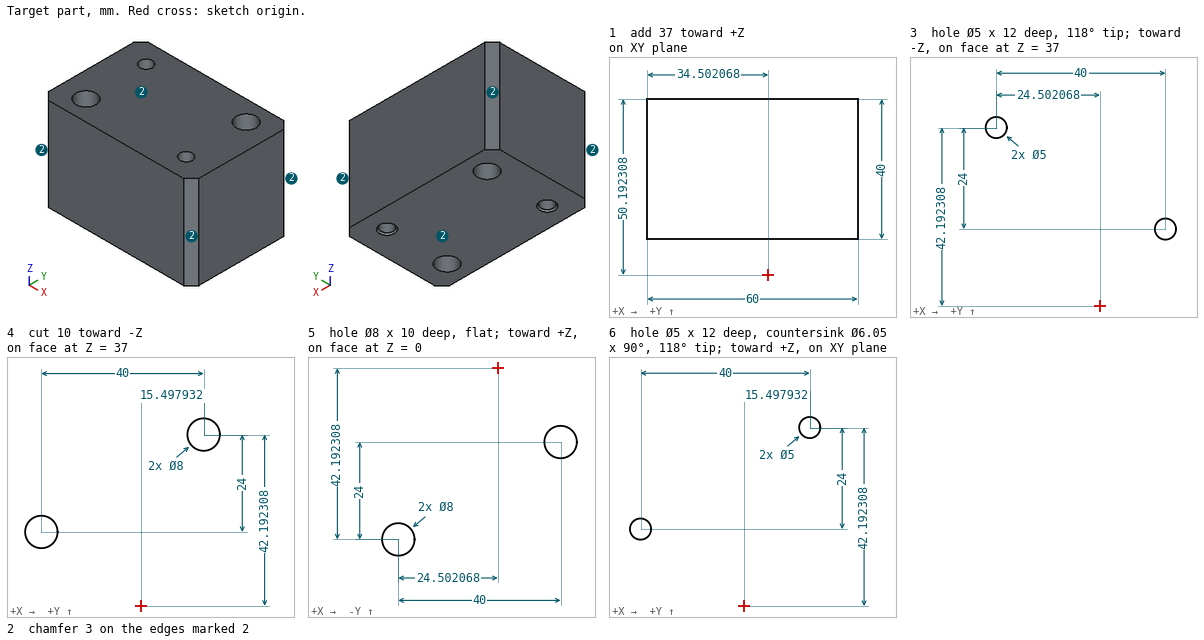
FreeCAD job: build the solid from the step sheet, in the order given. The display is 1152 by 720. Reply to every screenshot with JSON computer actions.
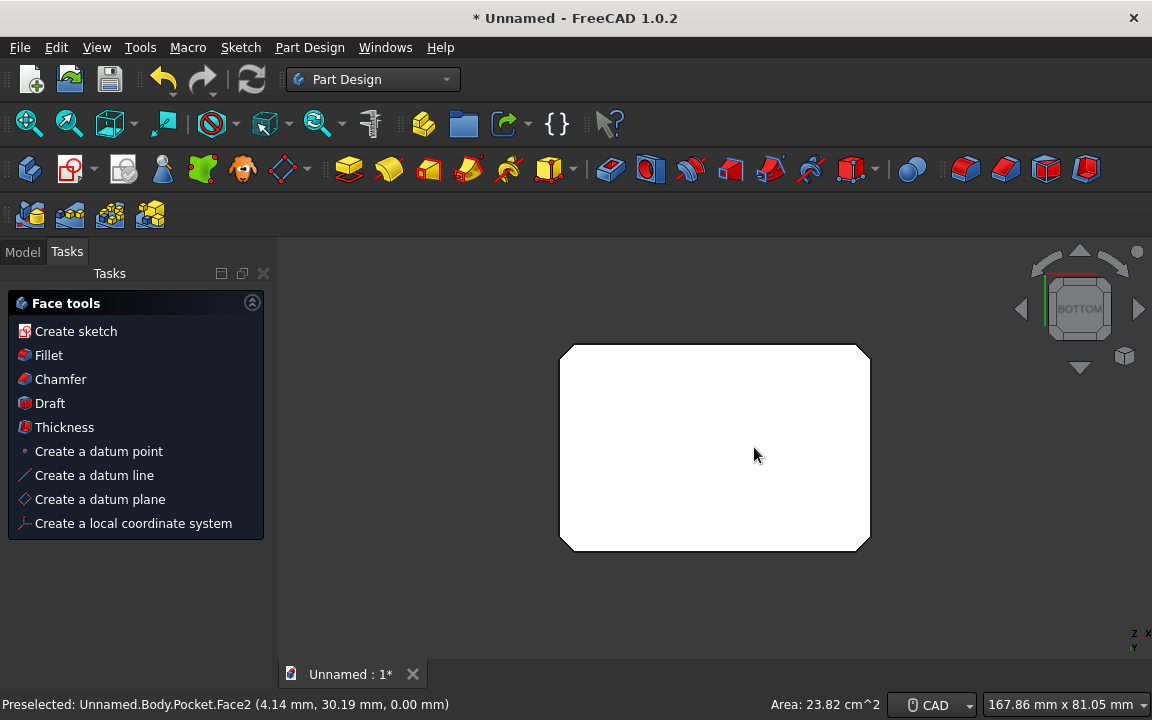
{"action": "left_click", "coordinate": [70, 170]}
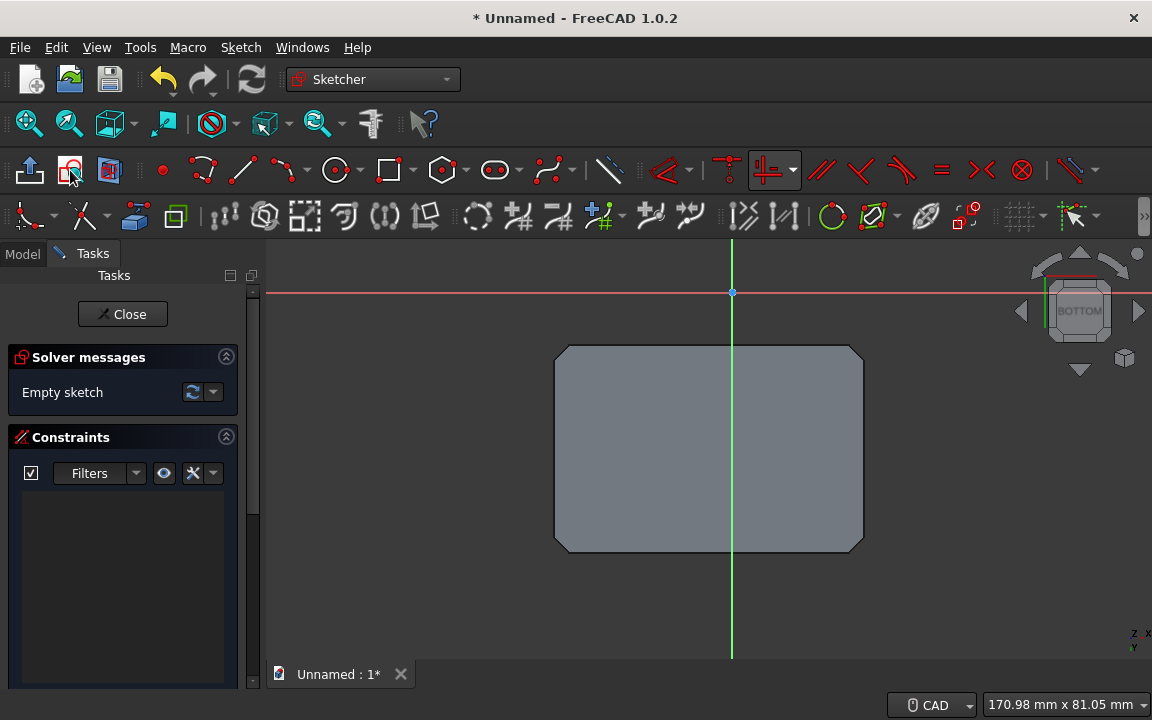
{"action": "left_click", "coordinate": [336, 170]}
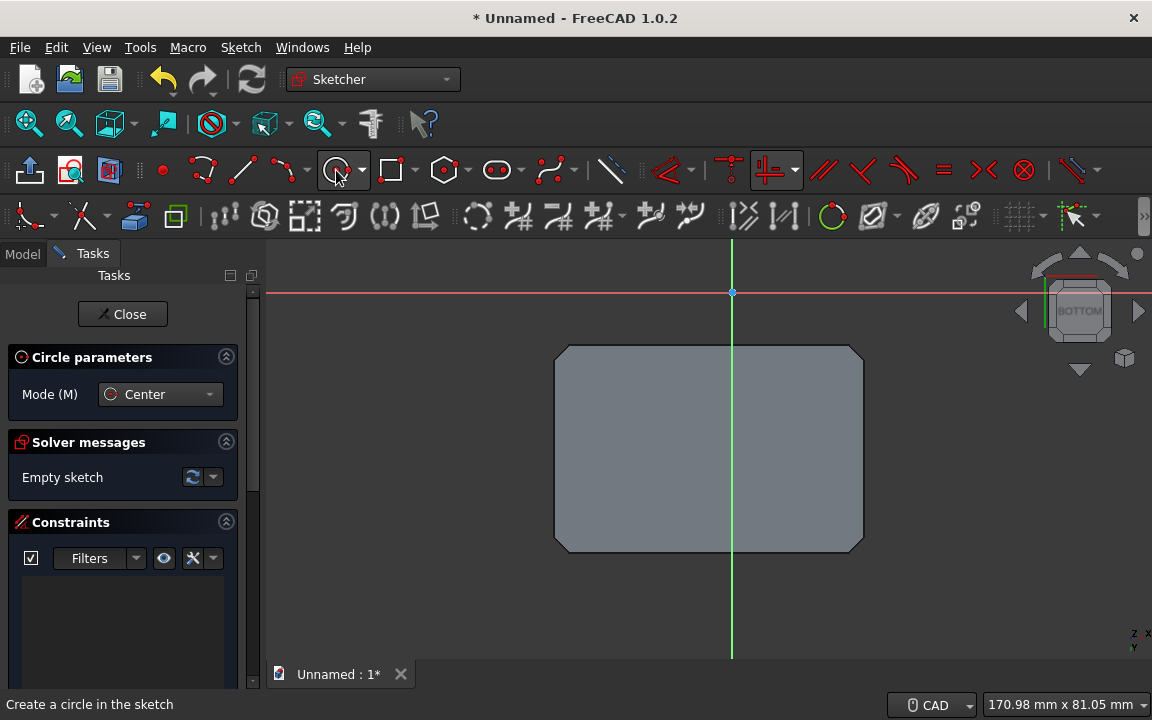
{"action": "left_click", "coordinate": [605, 511]}
{"action": "mouse_move", "coordinate": [620, 497]}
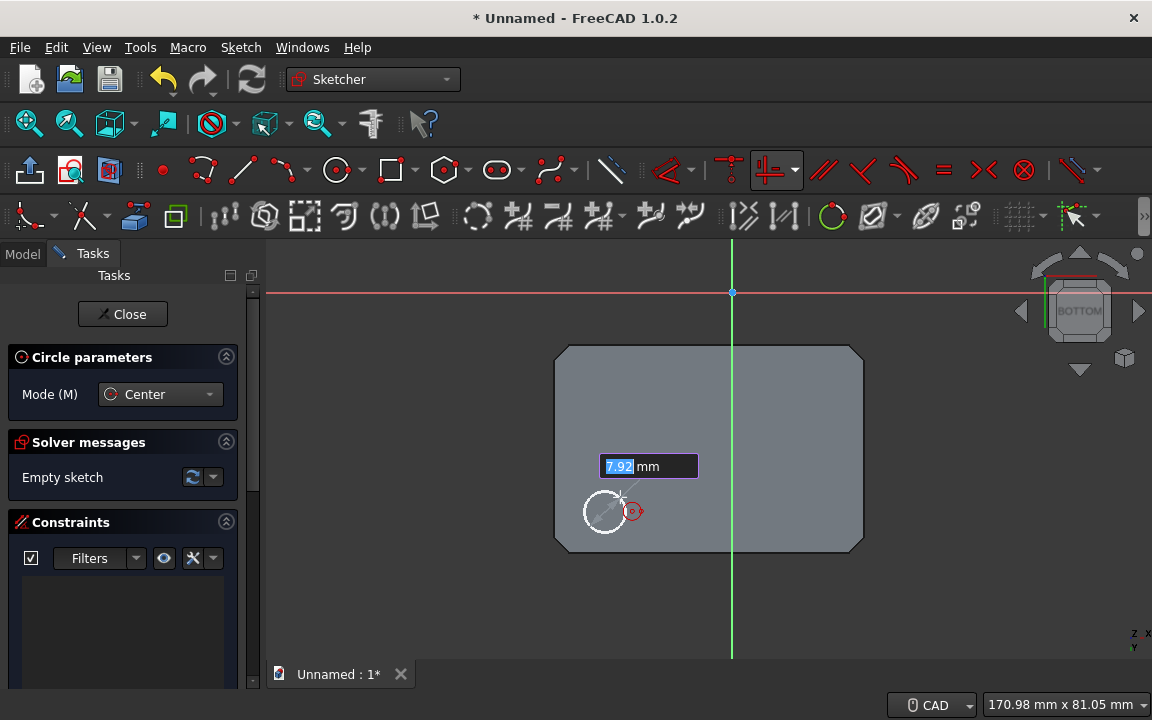
{"action": "type", "text": "8"}
{"action": "key", "text": "Return"}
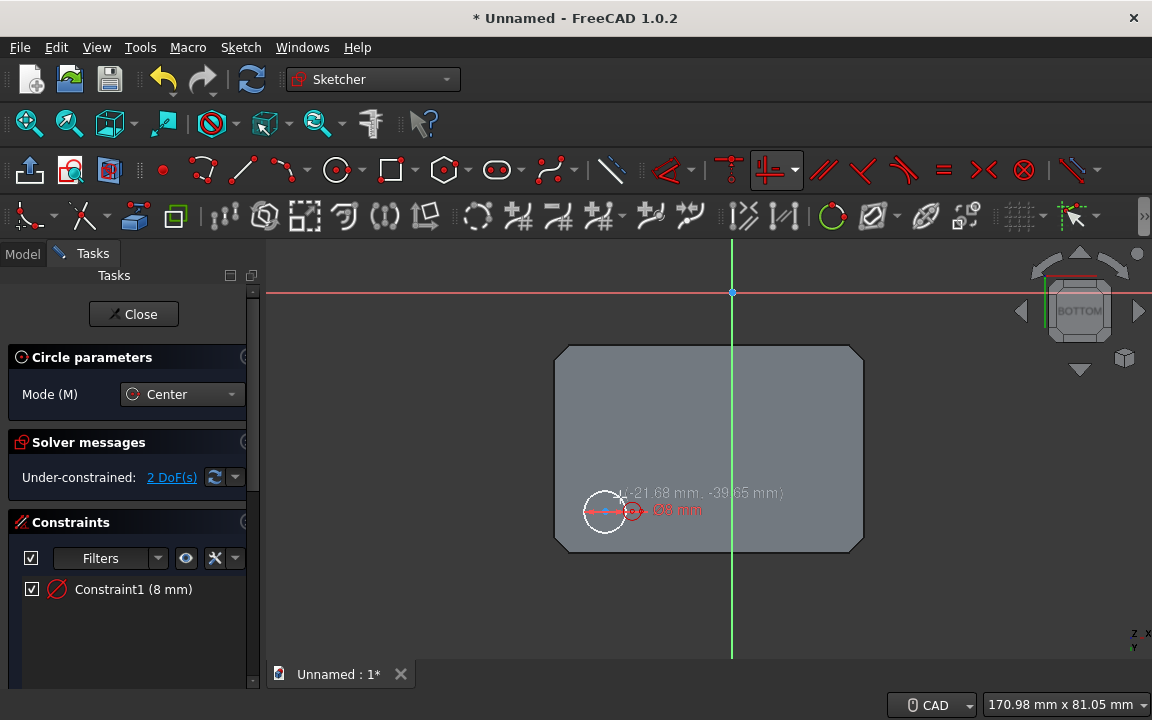
{"action": "left_click", "coordinate": [813, 387]}
{"action": "mouse_move", "coordinate": [827, 372]}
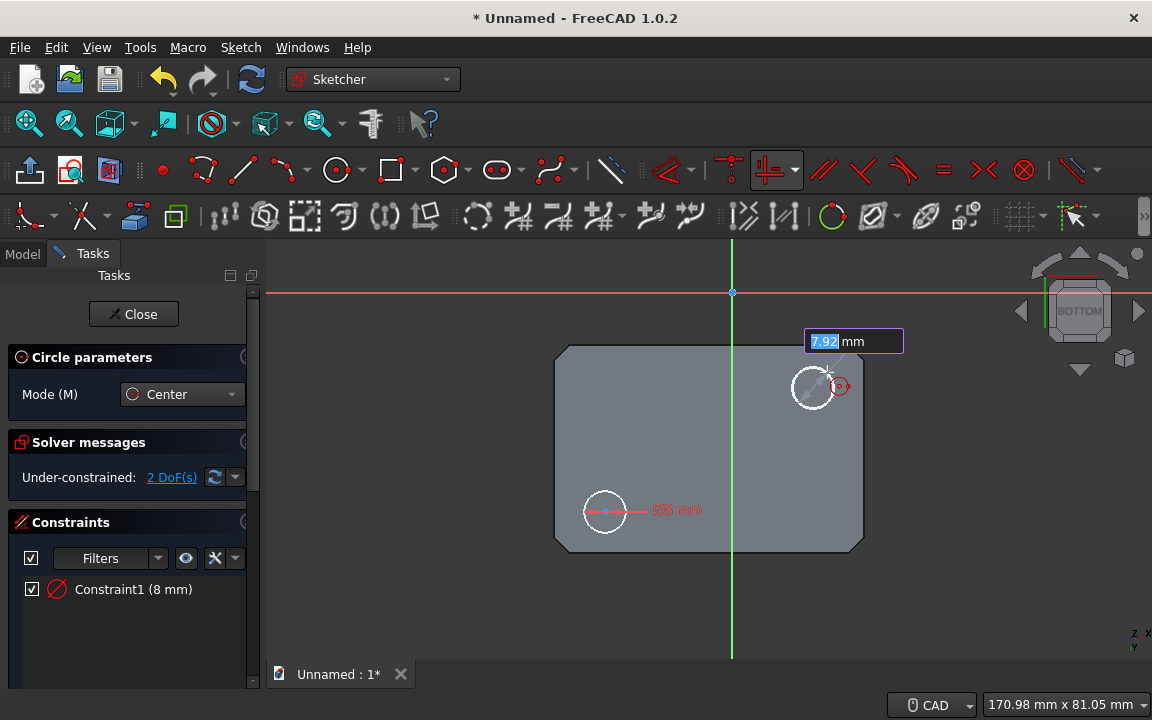
{"action": "type", "text": "8"}
{"action": "key", "text": "Return"}
{"action": "key", "text": "Escape"}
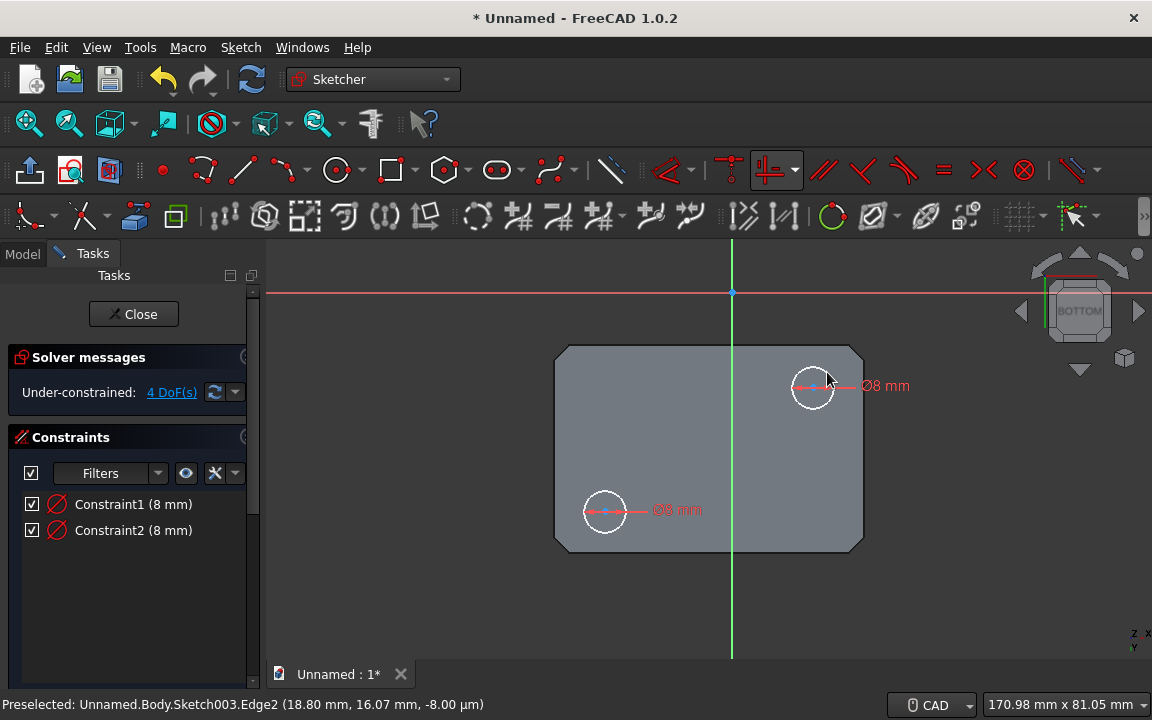
{"action": "left_click", "coordinate": [666, 170]}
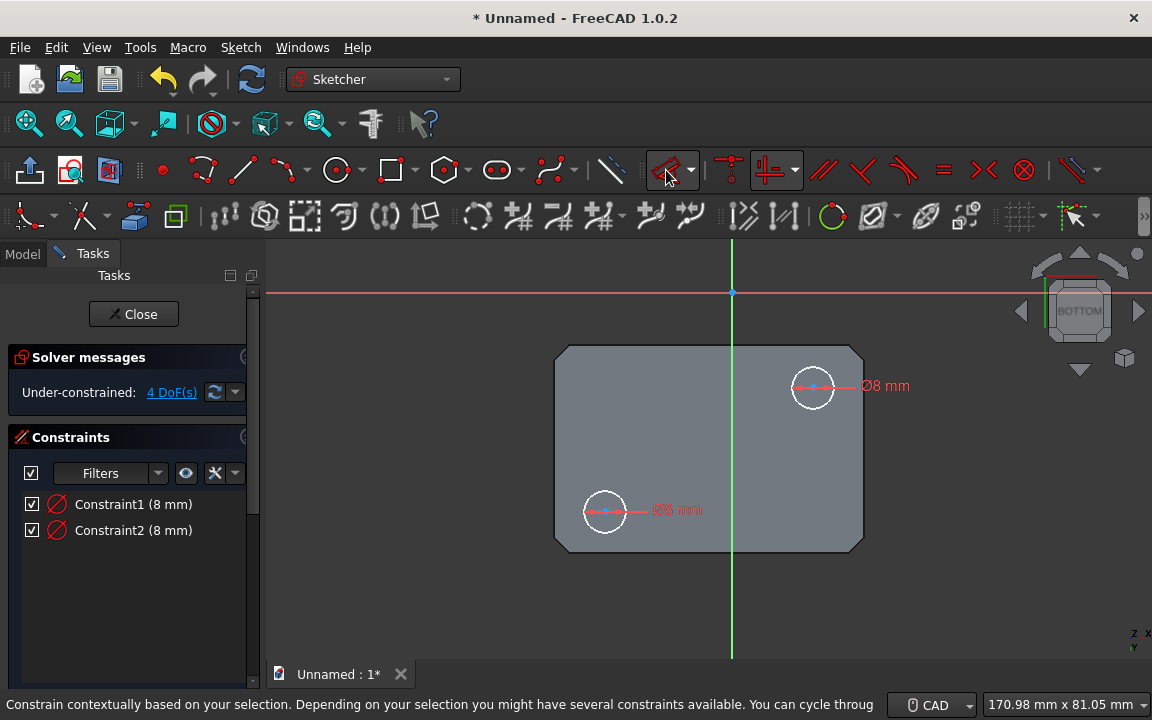
{"action": "left_click", "coordinate": [605, 512]}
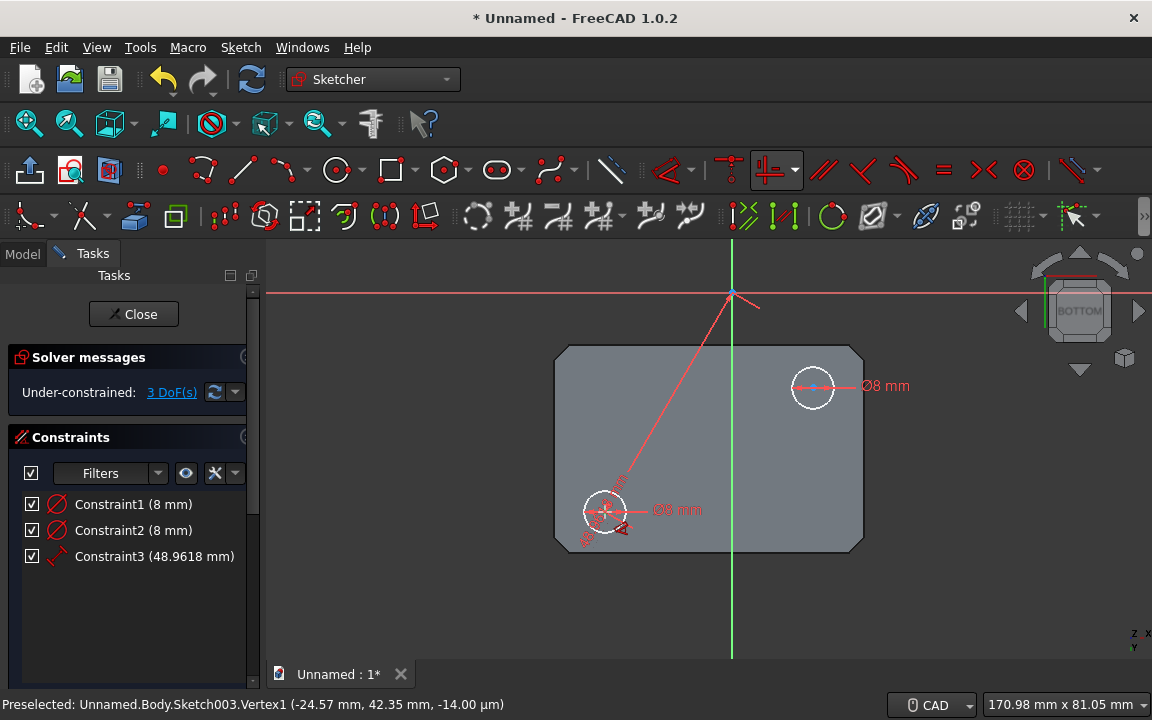
{"action": "left_click", "coordinate": [813, 388]}
{"action": "left_click", "coordinate": [709, 546]}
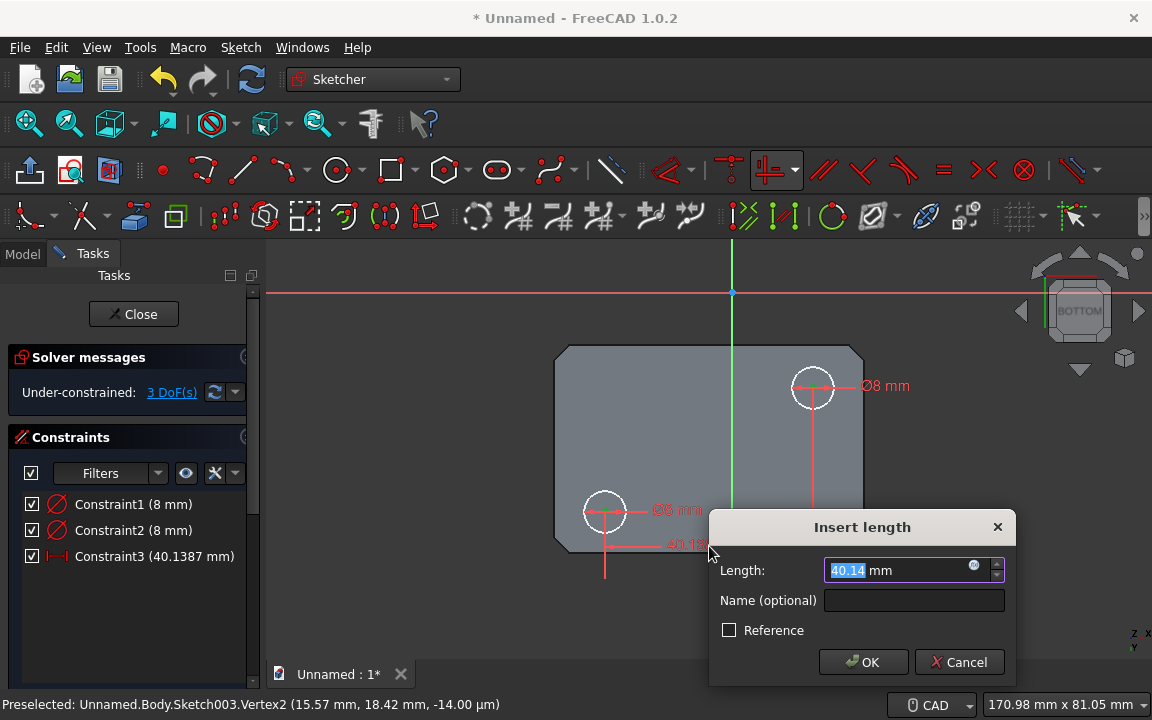
{"action": "type", "text": "40"}
{"action": "key", "text": "Return"}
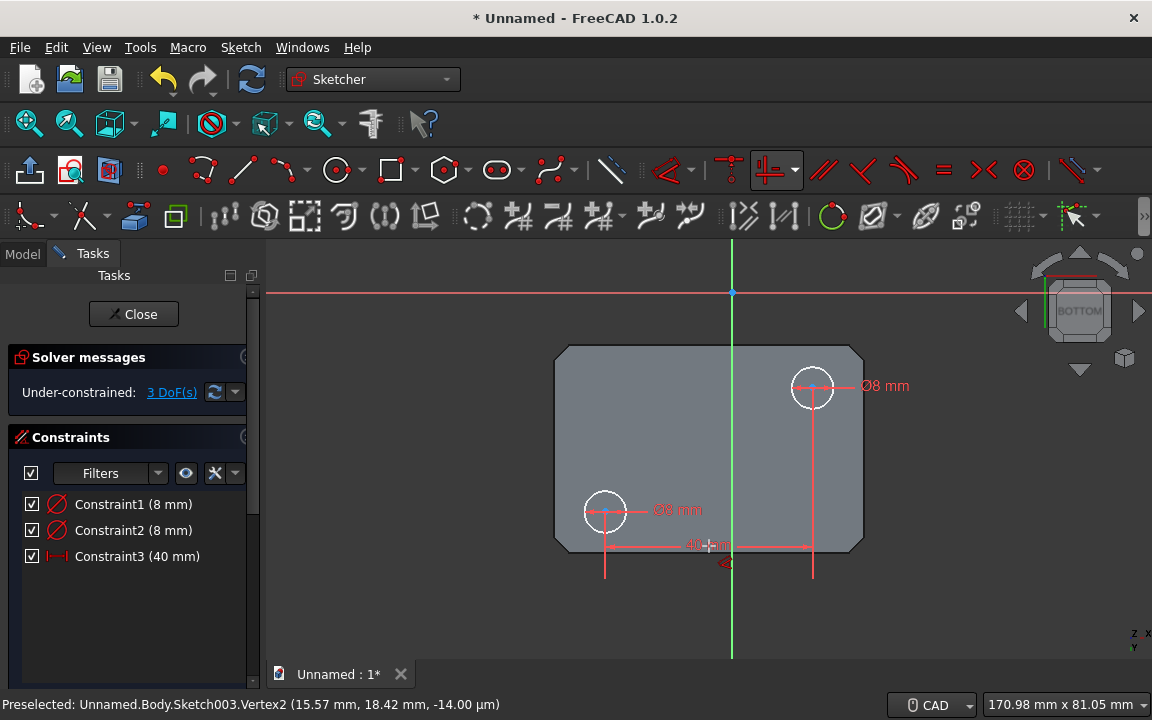
{"action": "left_click", "coordinate": [605, 512]}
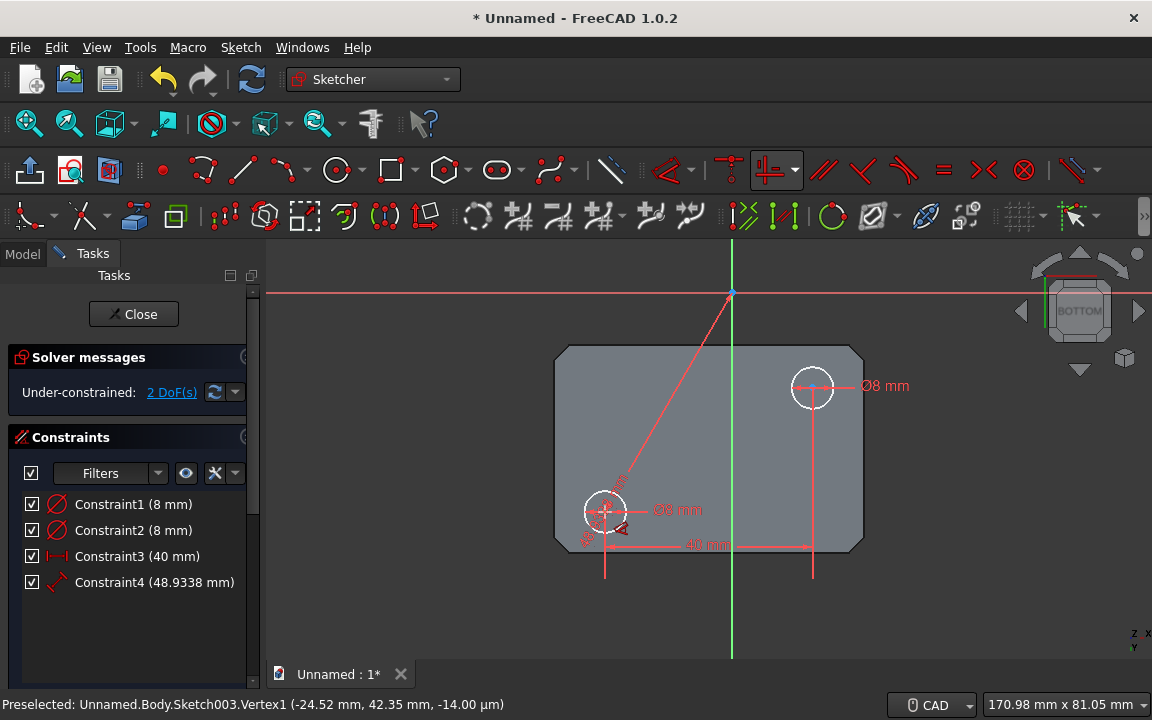
{"action": "left_click", "coordinate": [813, 388]}
{"action": "left_click", "coordinate": [571, 450]}